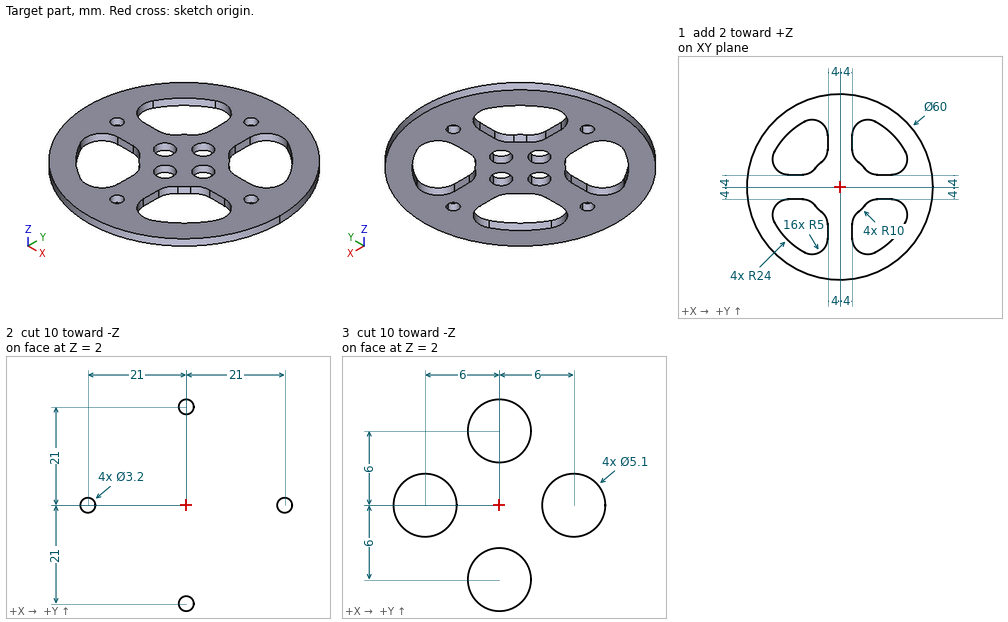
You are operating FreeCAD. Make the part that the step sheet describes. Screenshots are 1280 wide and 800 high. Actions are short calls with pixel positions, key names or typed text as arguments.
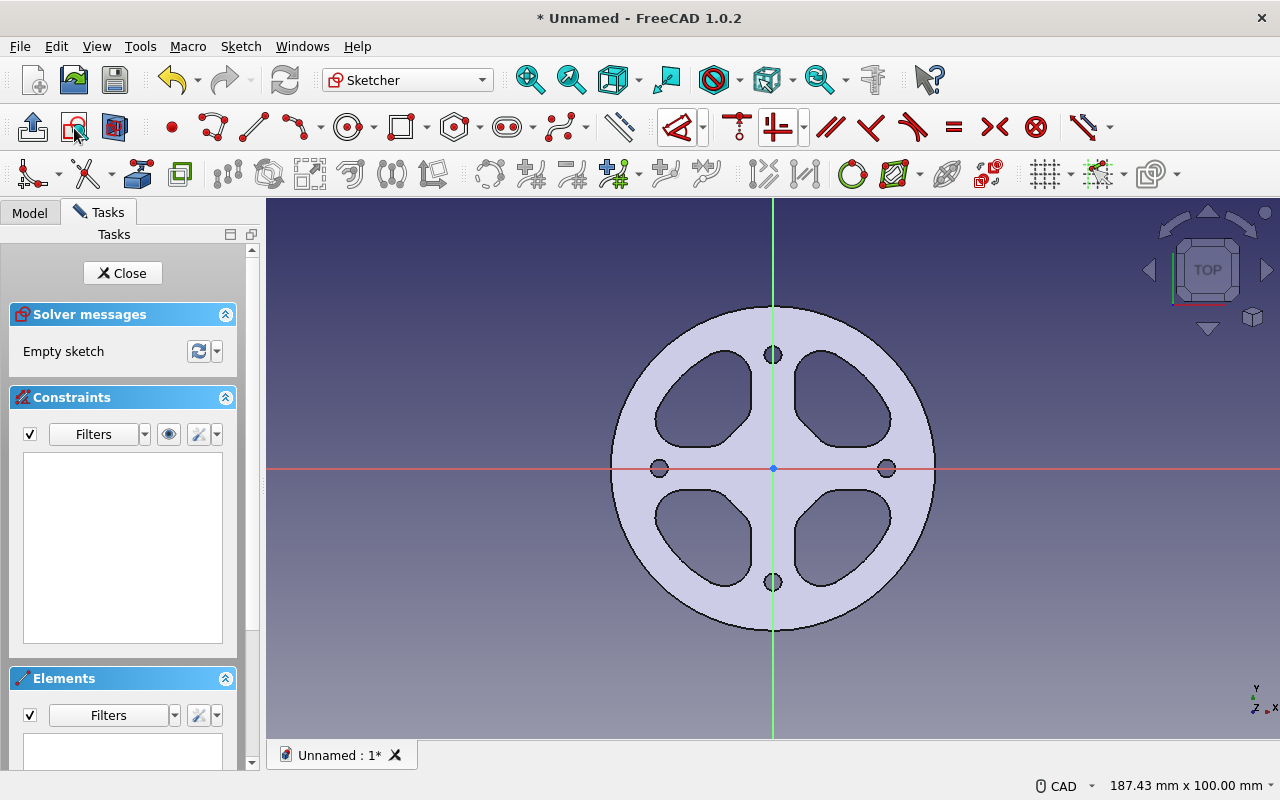
scroll(795, 468, up, 7)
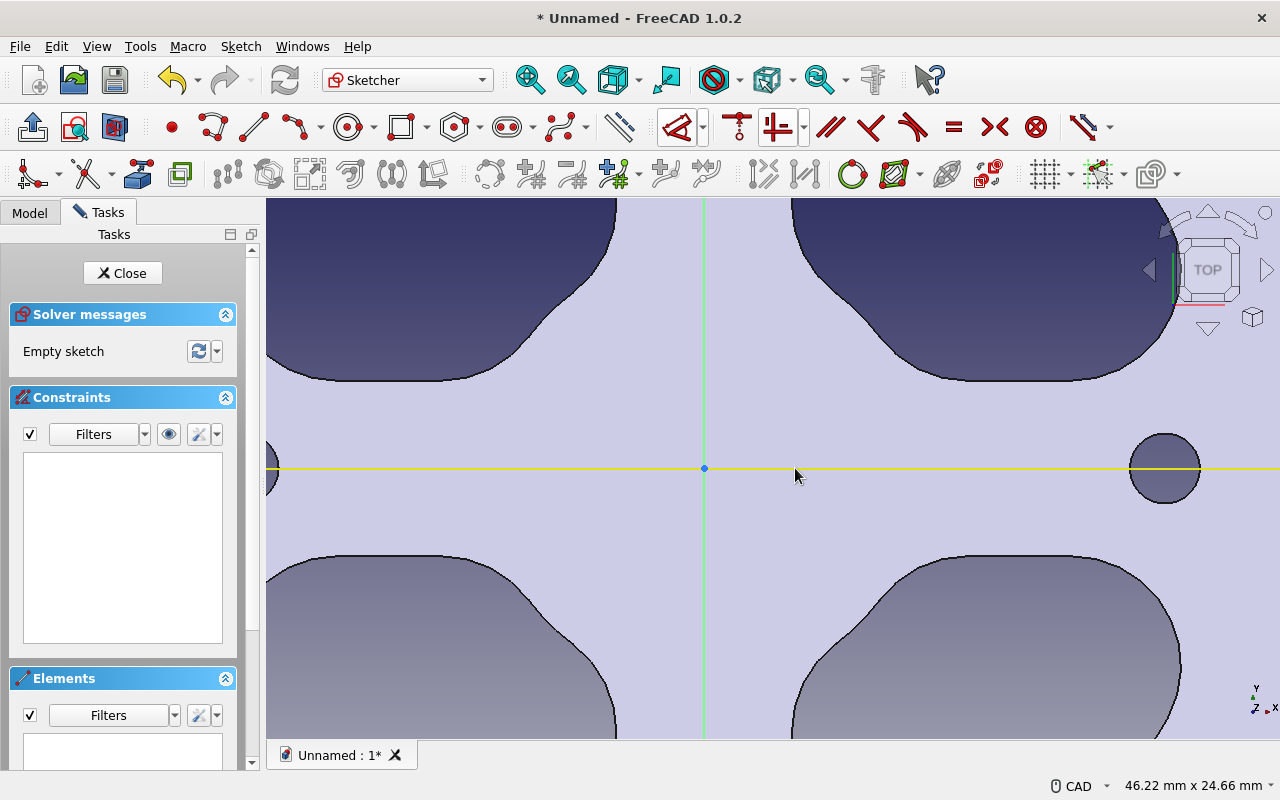
click(348, 128)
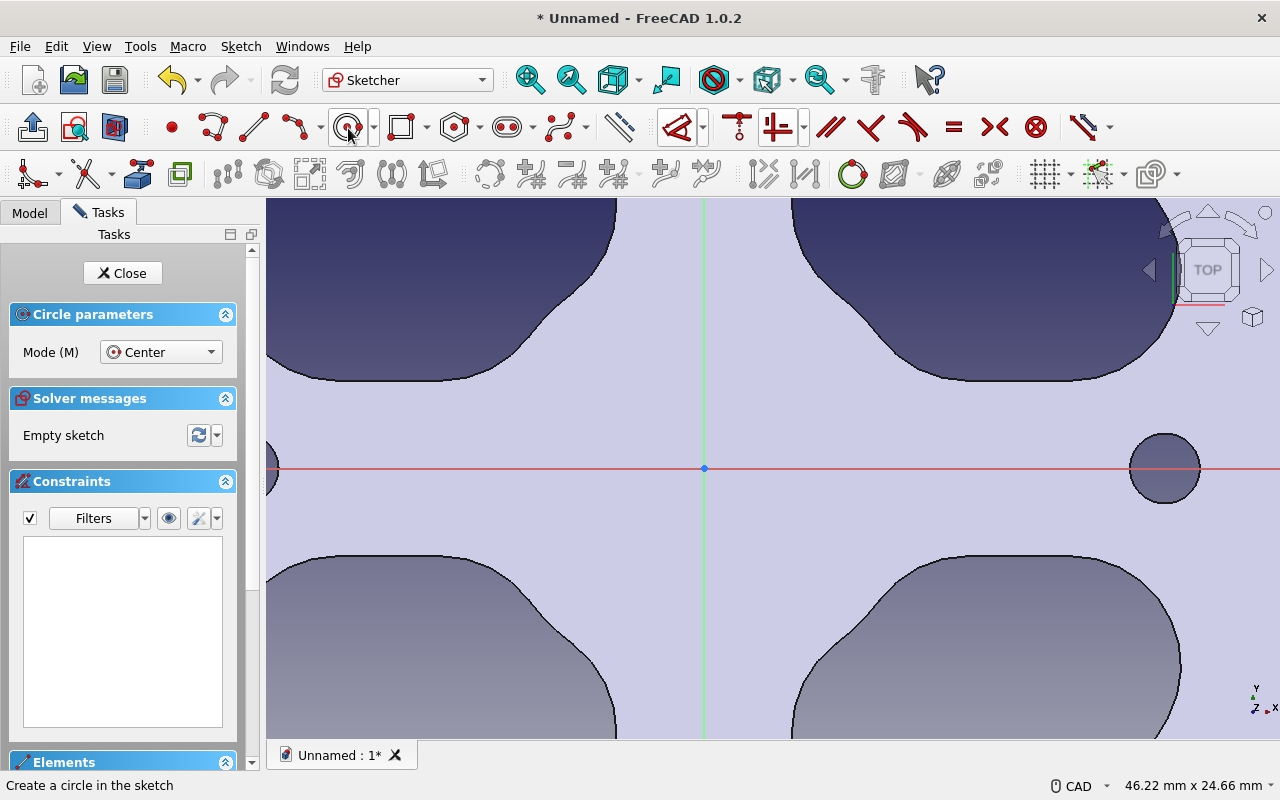
click(704, 337)
move(744, 297)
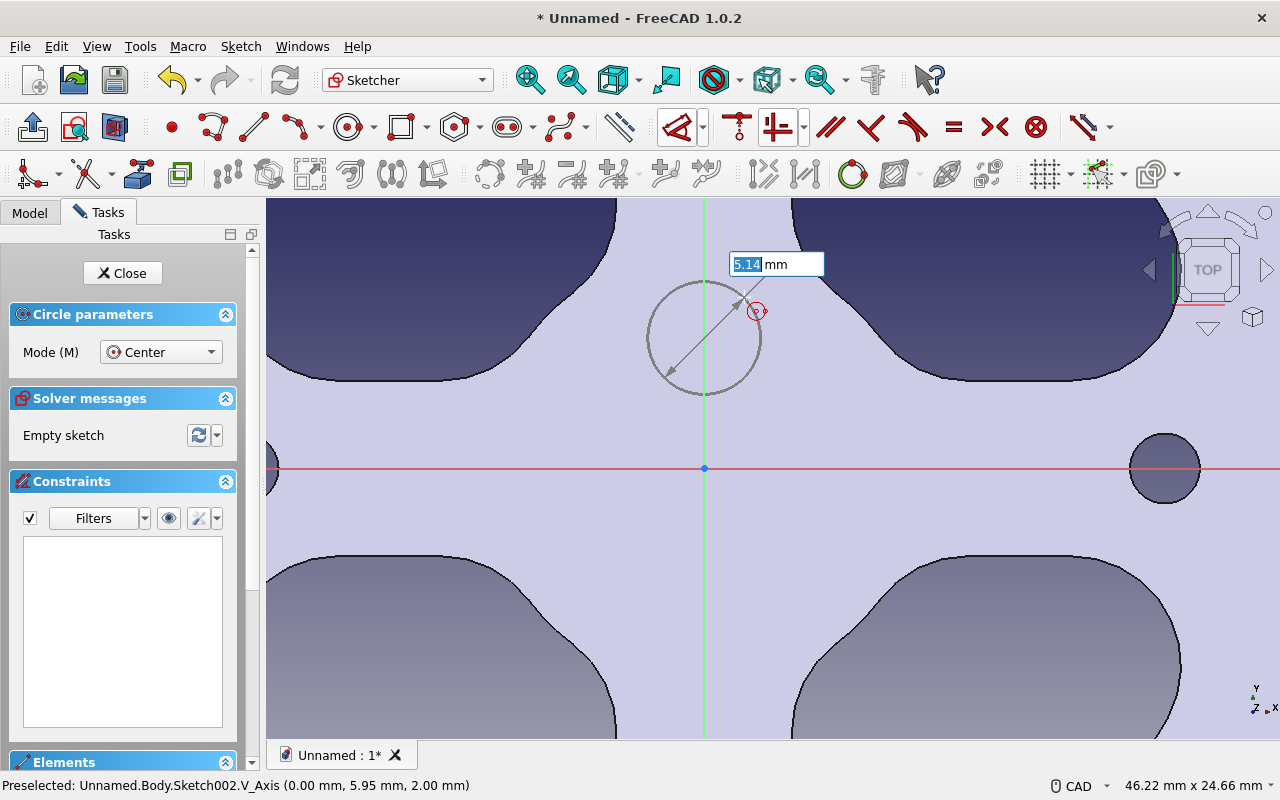
text(5.1)
key(Return)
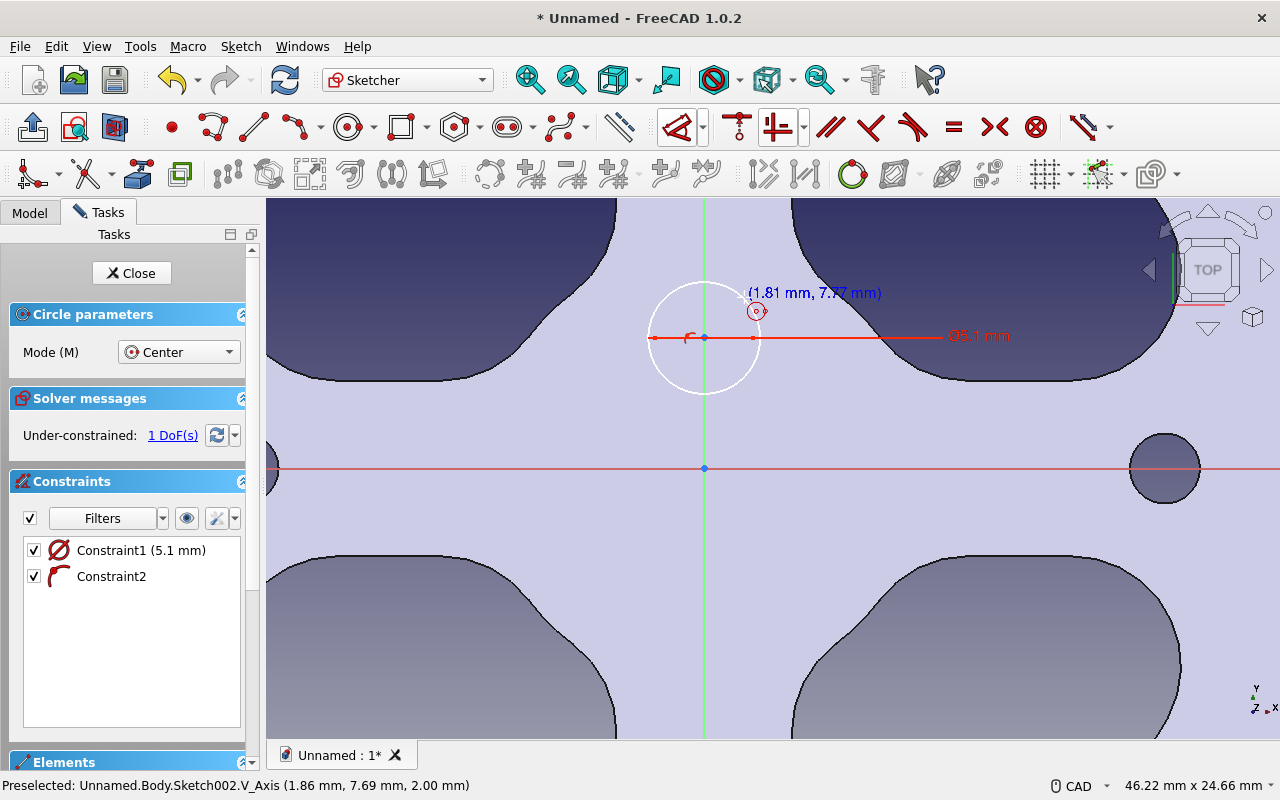
click(573, 468)
move(612, 429)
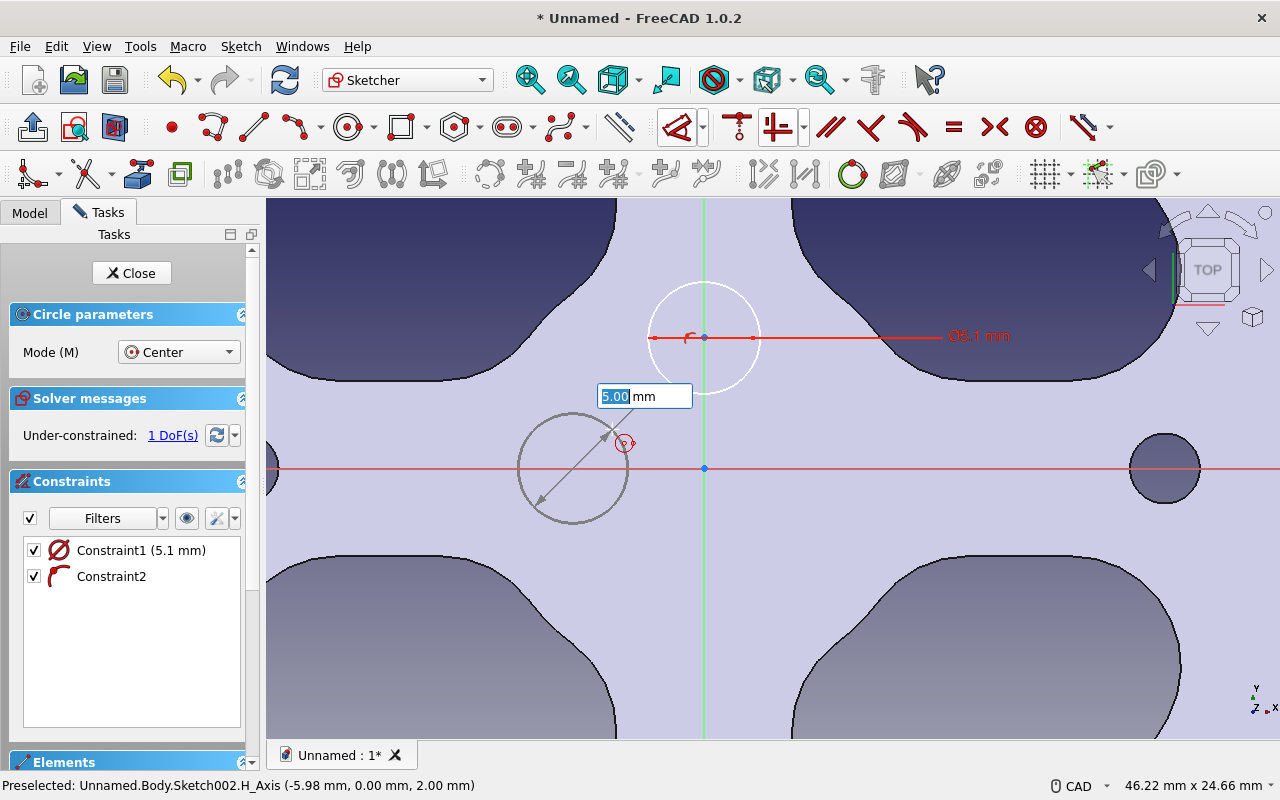
text(5.1)
key(Return)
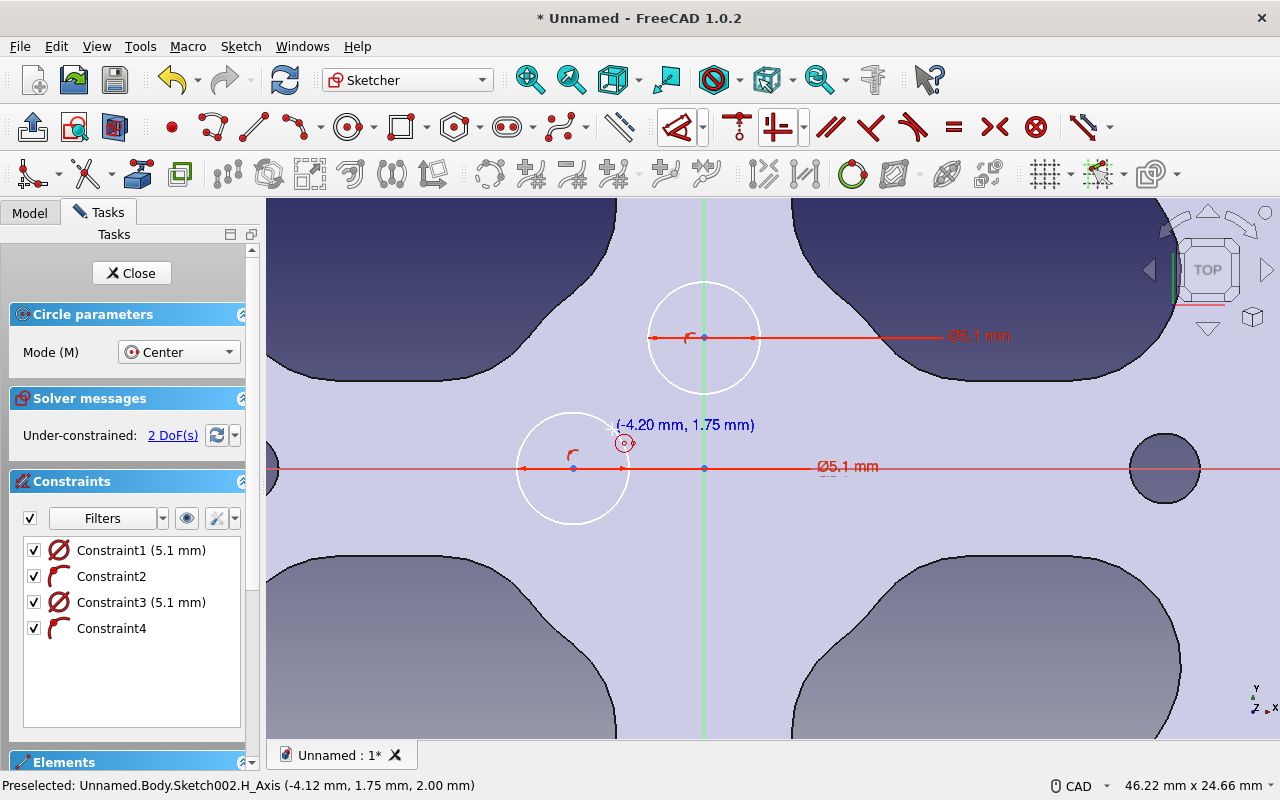
click(836, 468)
move(875, 429)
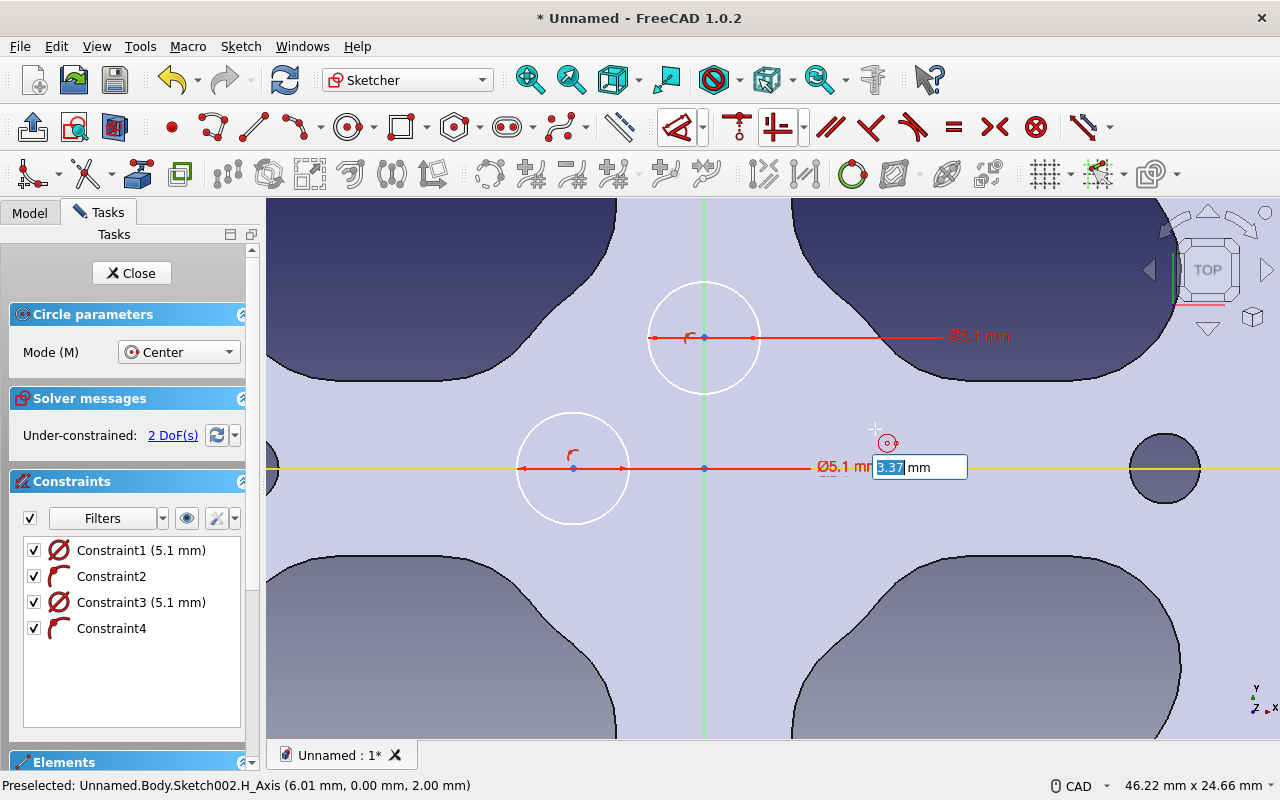
text(5.1)
key(Return)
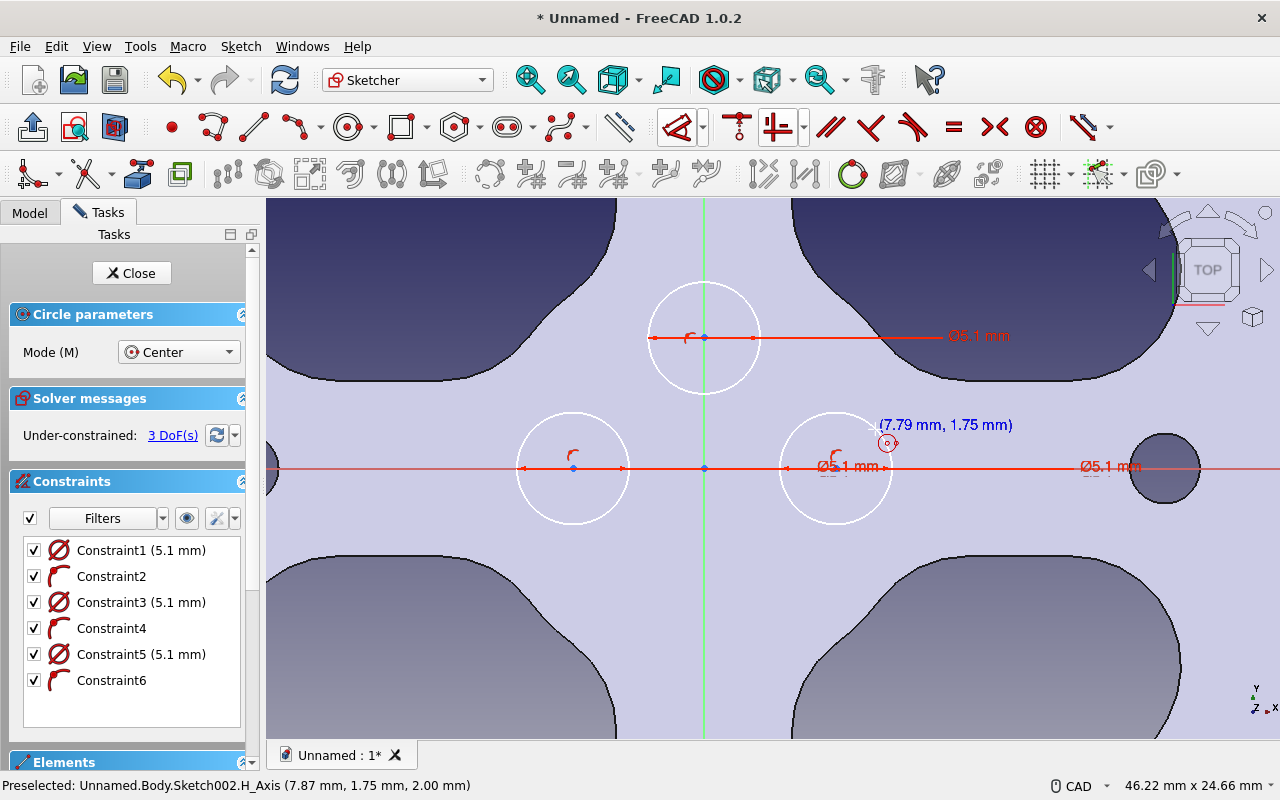
click(704, 600)
move(744, 561)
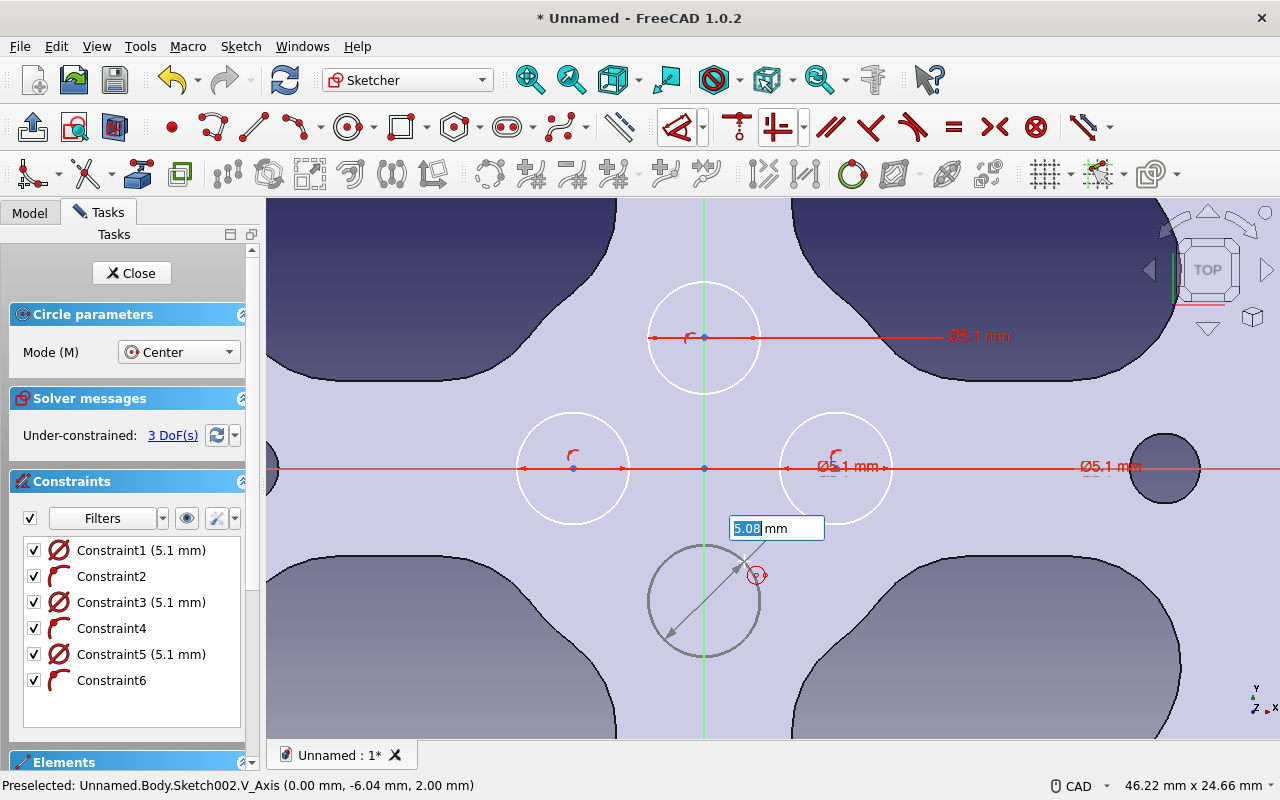
text(5.1)
key(Return)
key(Escape)